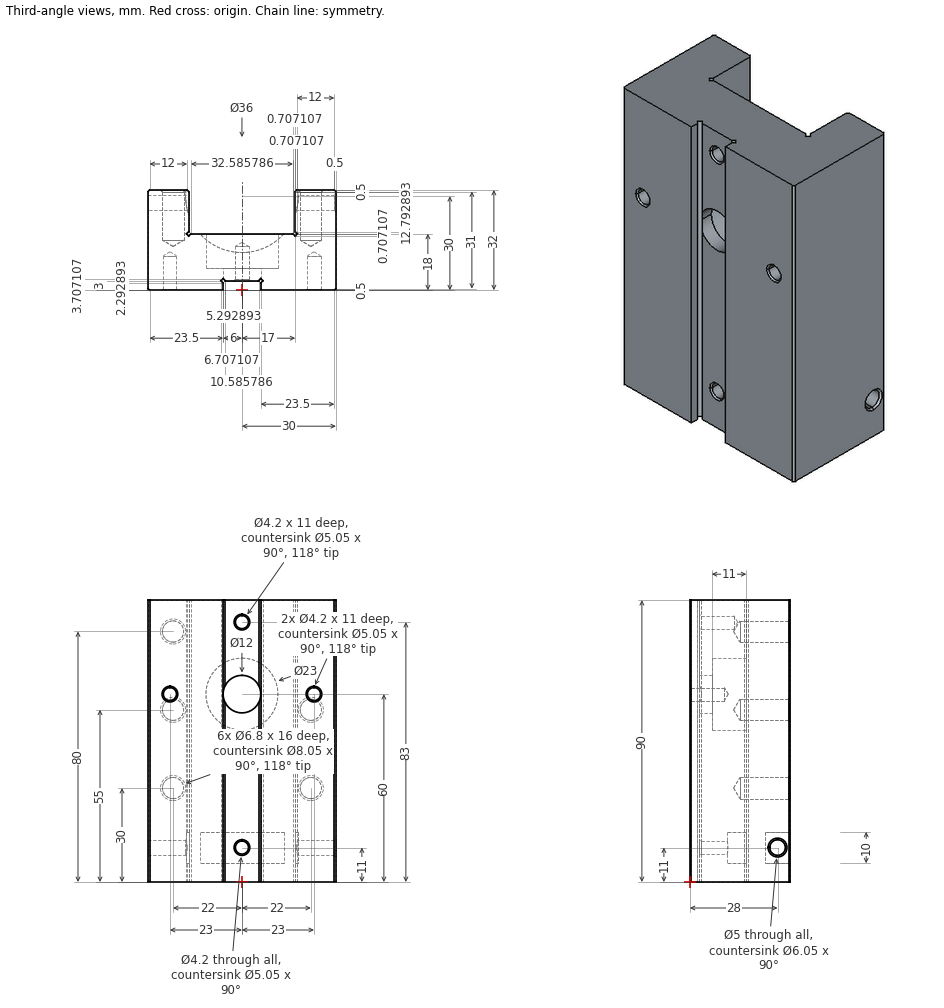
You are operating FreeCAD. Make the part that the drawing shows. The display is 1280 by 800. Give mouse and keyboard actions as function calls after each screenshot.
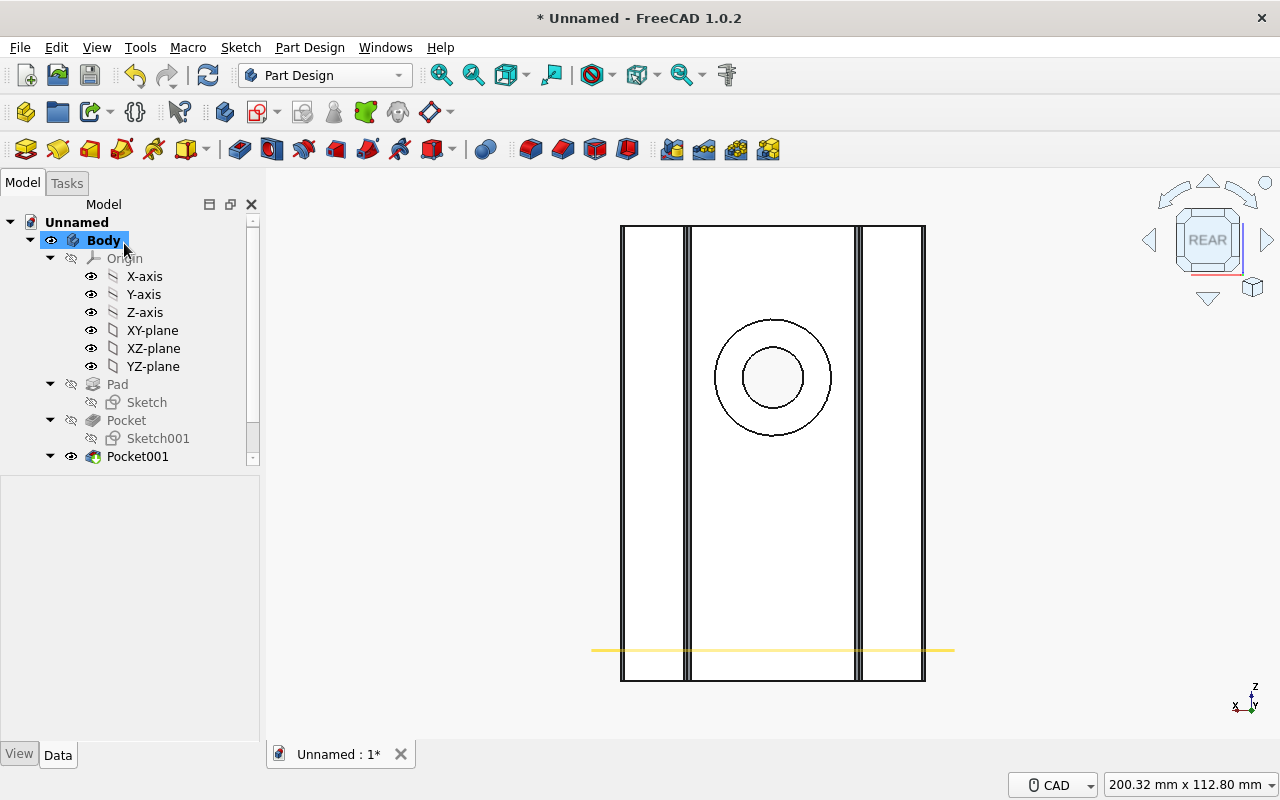
scroll(100, 344, down, 3)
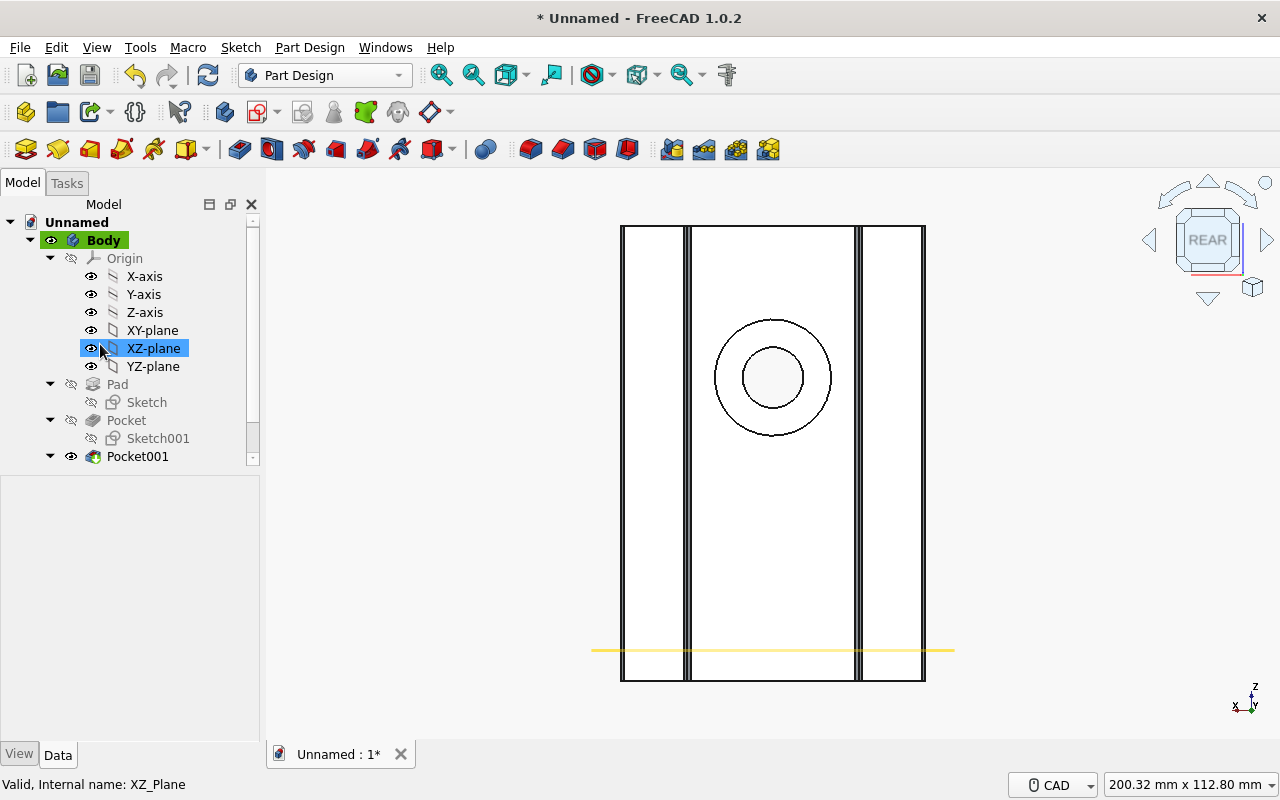
click(116, 456)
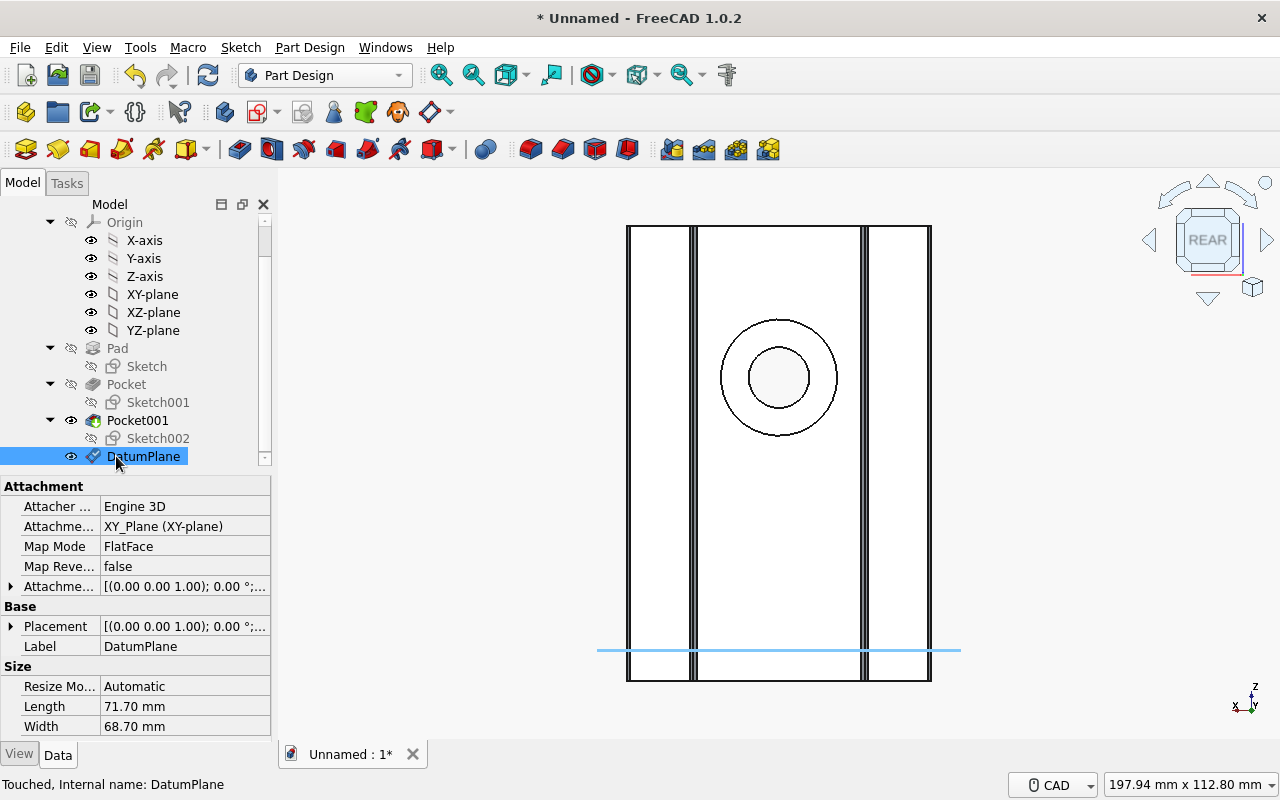
click(258, 112)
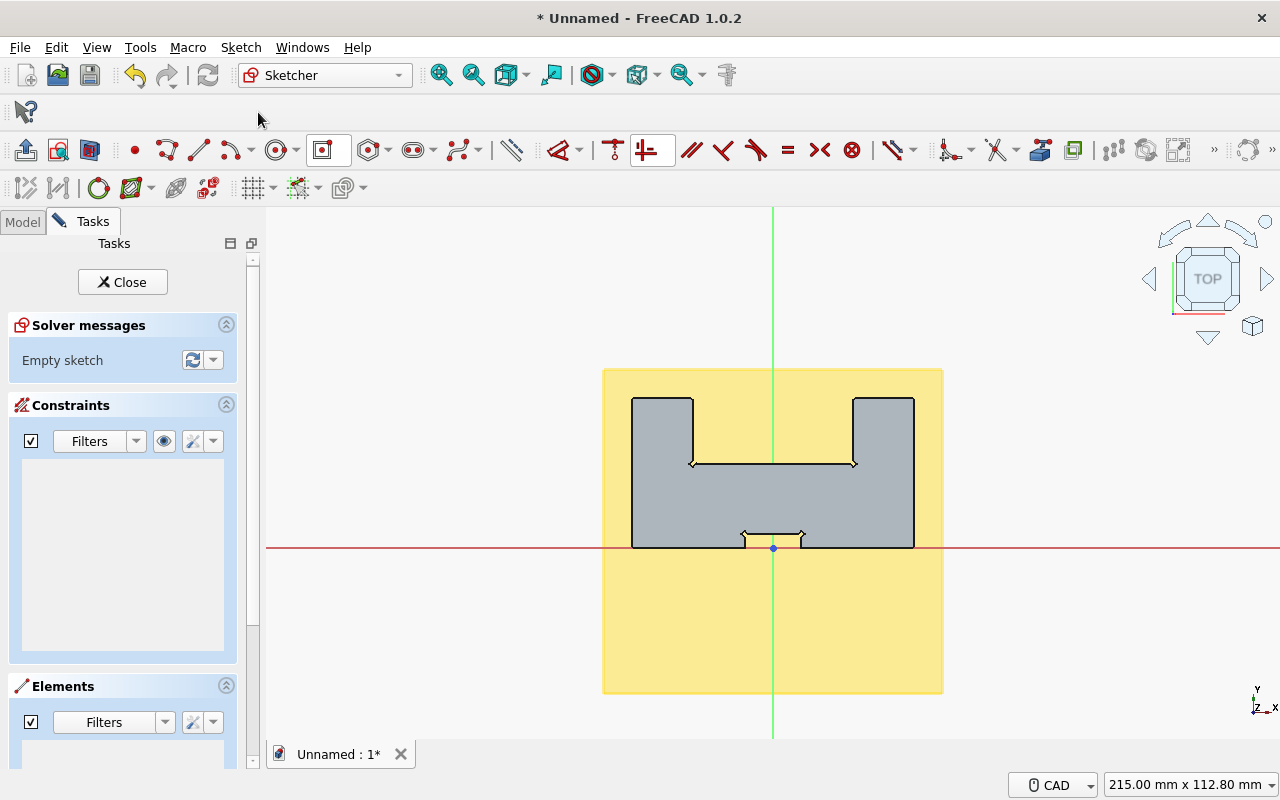
click(90, 150)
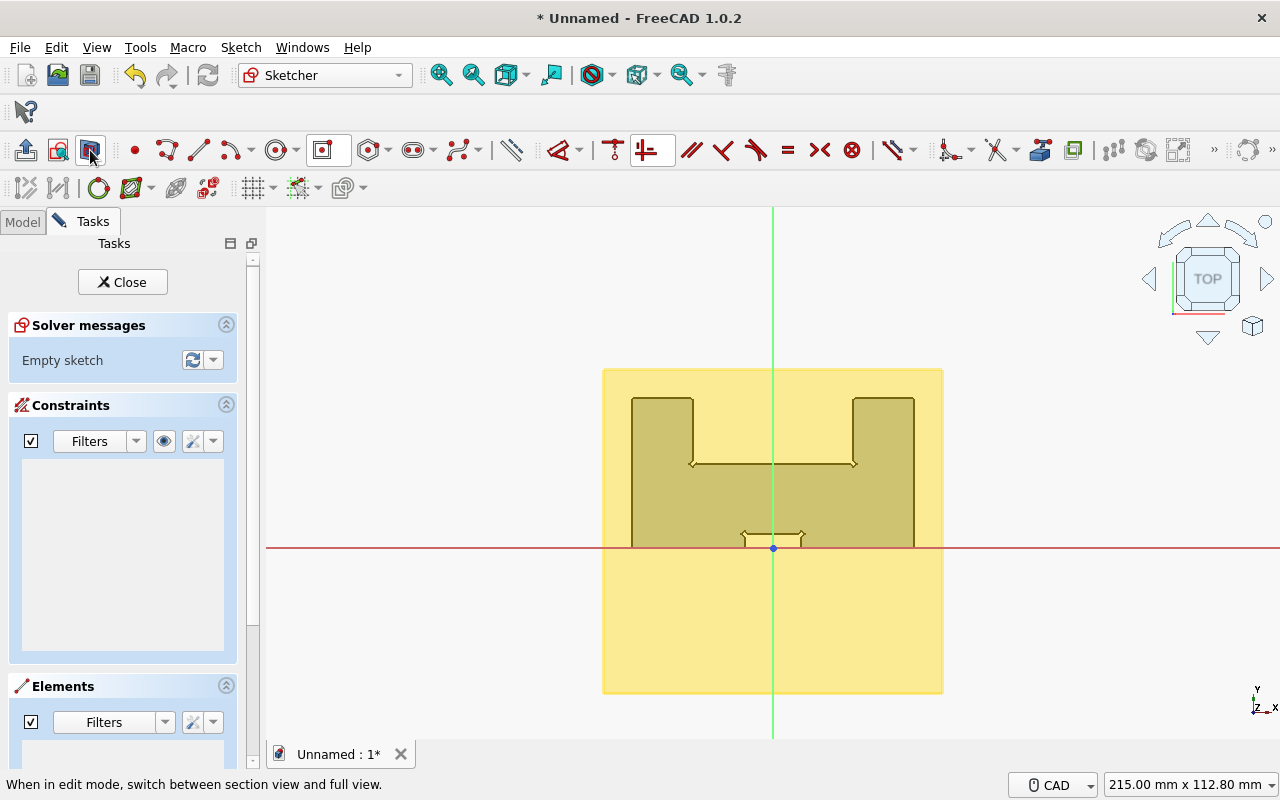
scroll(912, 359, up, 2)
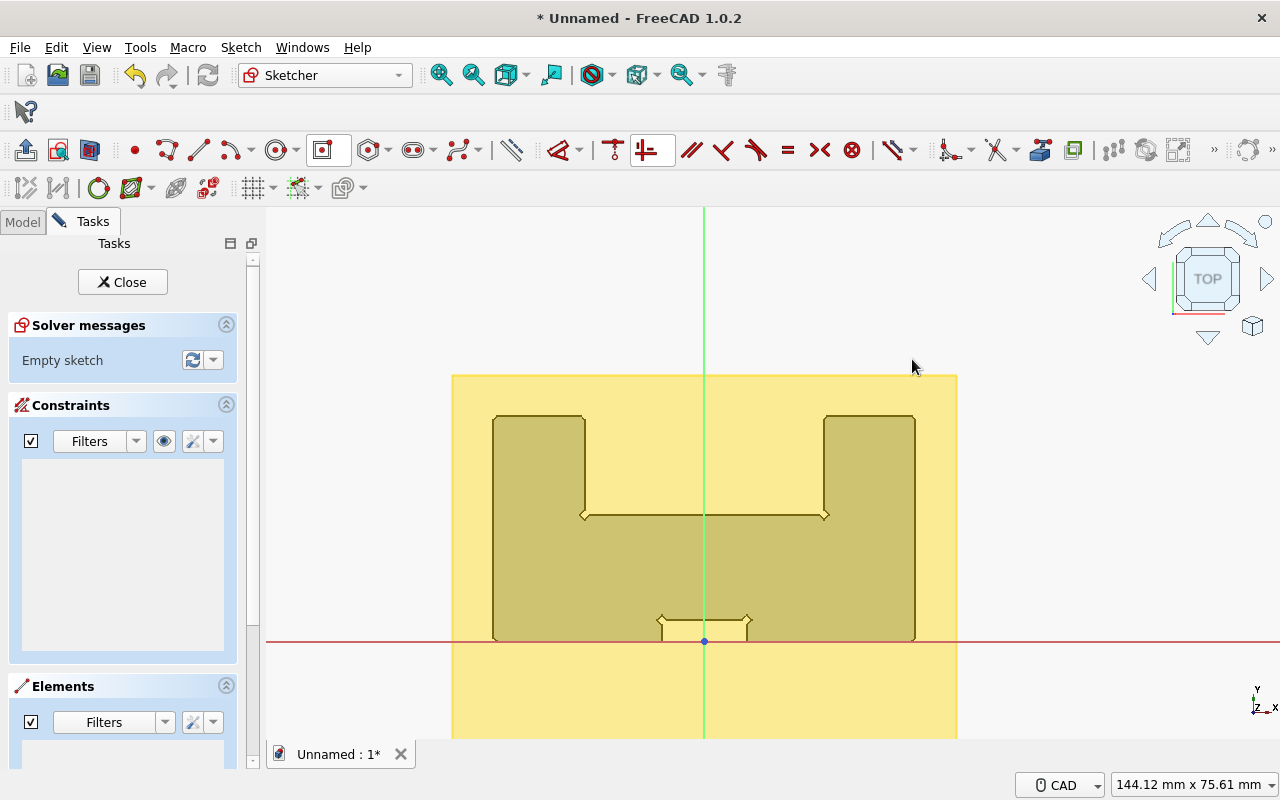
click(276, 150)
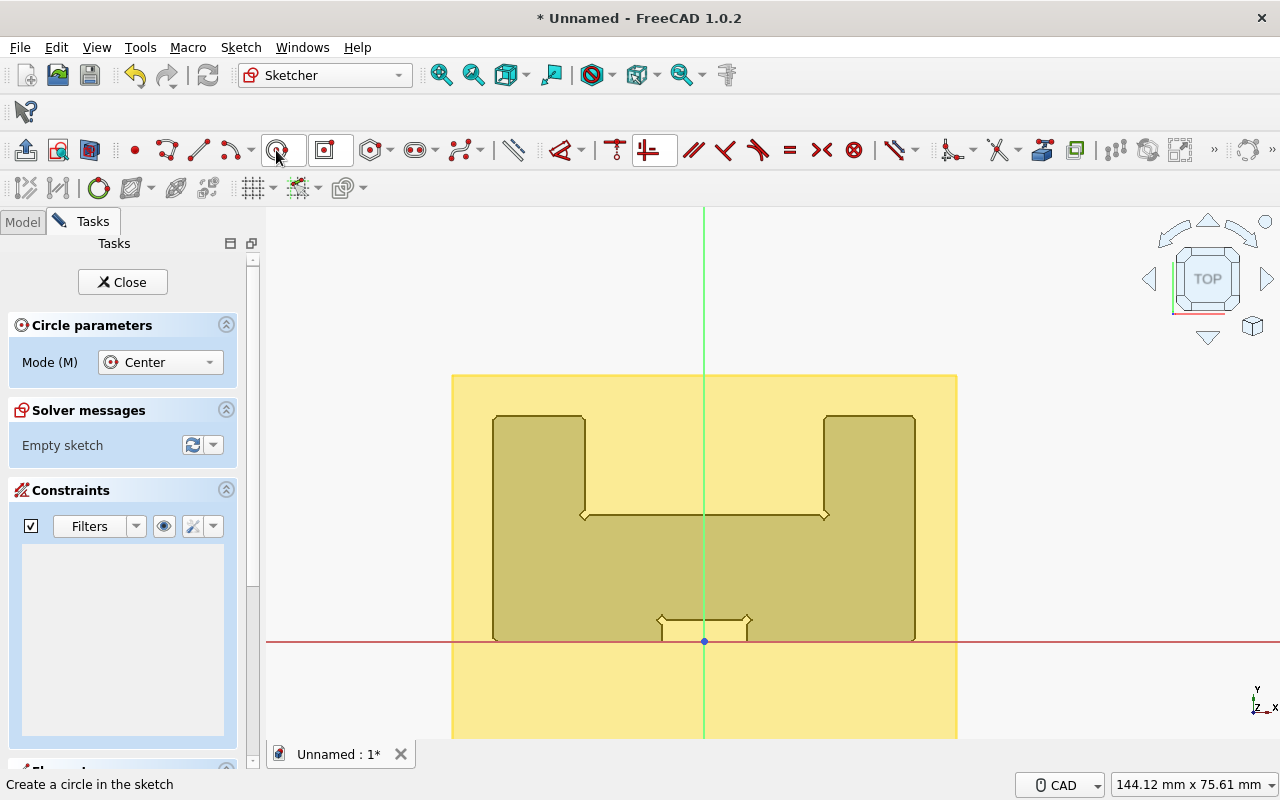
click(704, 430)
move(794, 341)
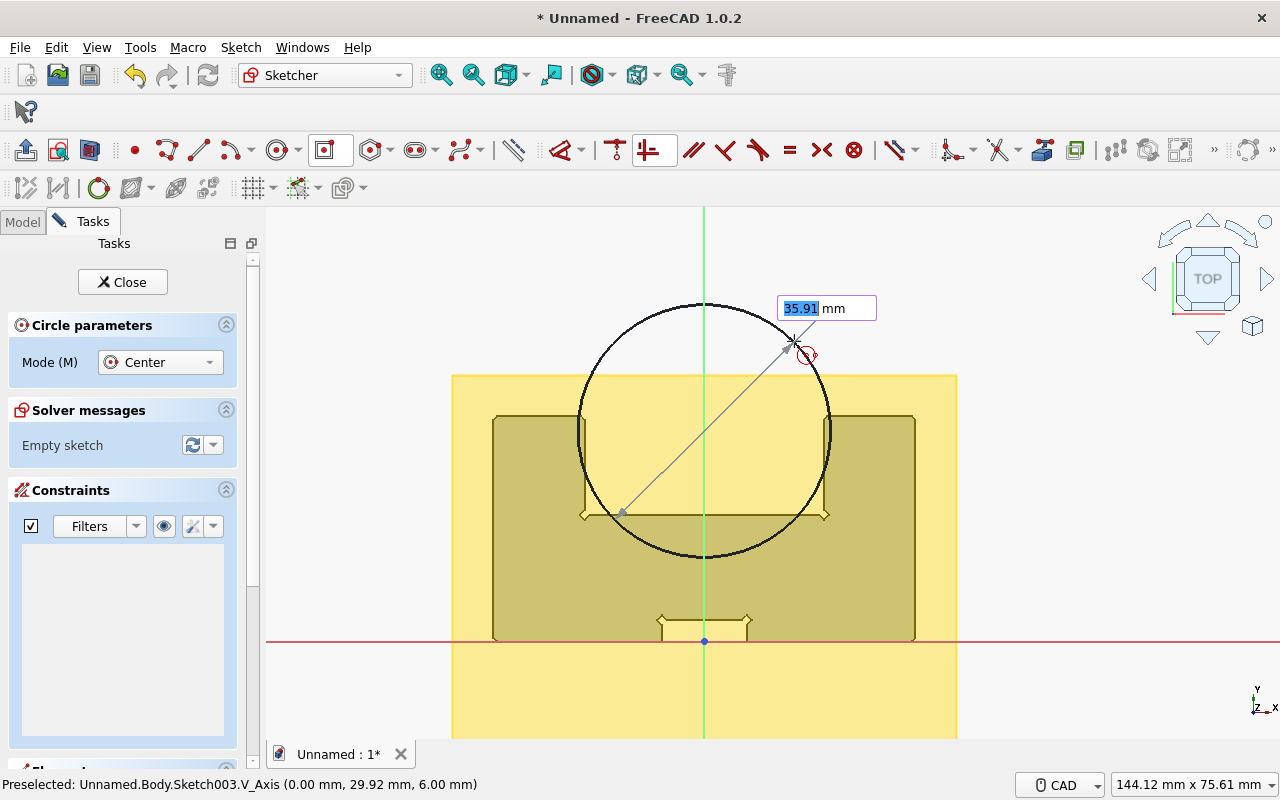
text(36)
key(Return)
key(Escape)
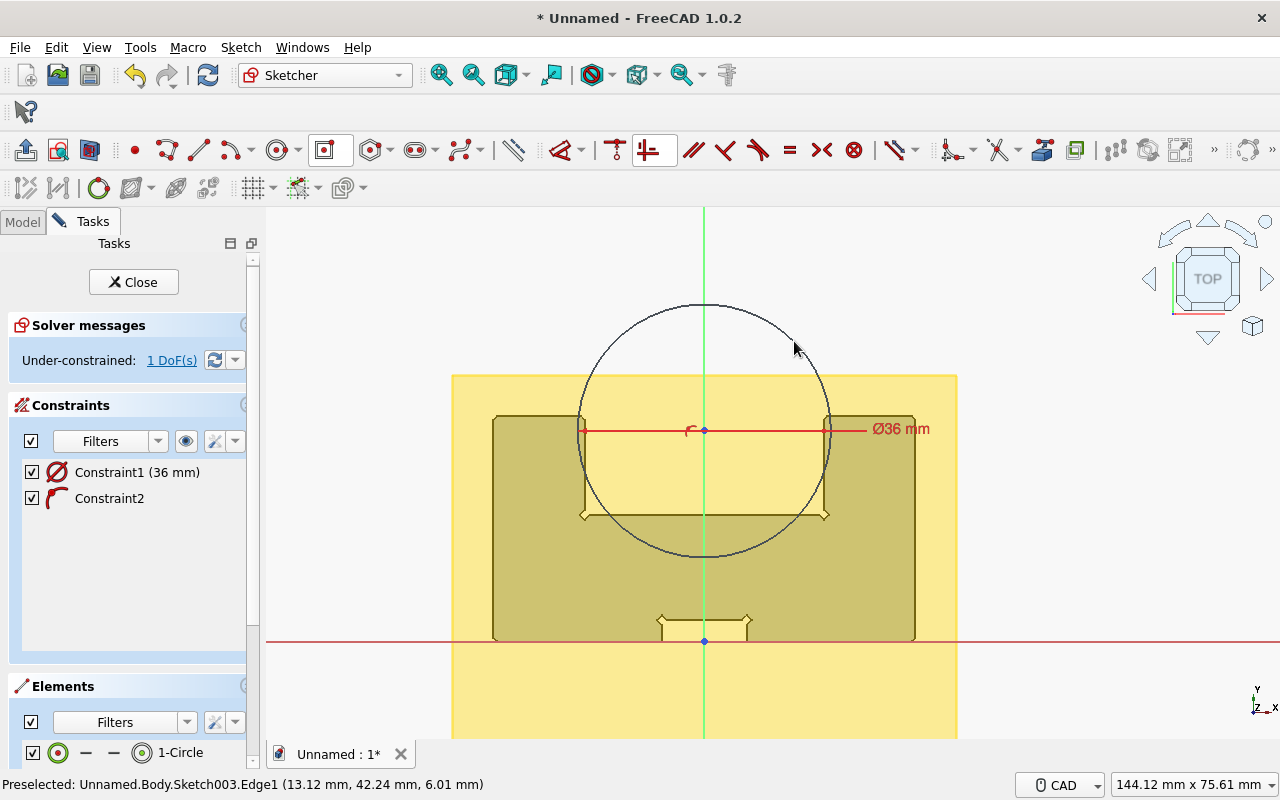
click(560, 150)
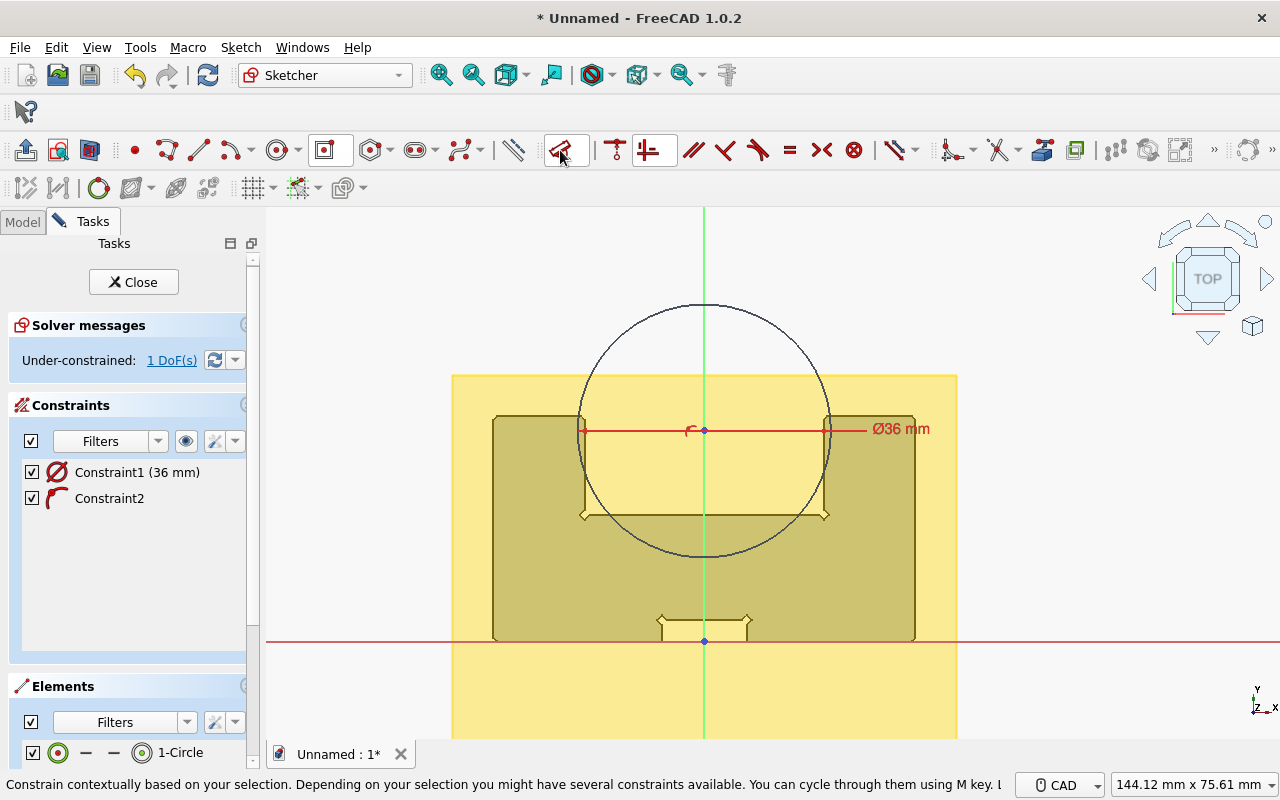
click(704, 431)
click(738, 536)